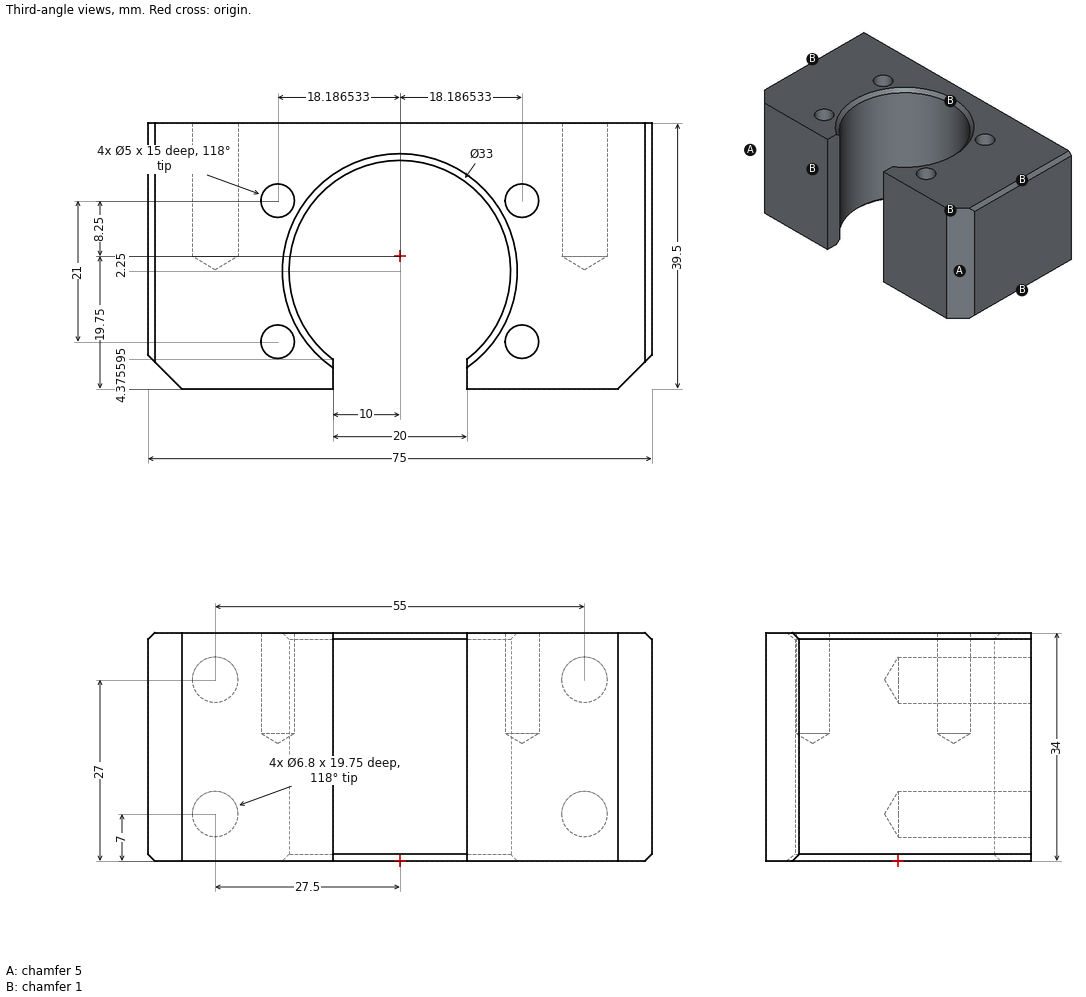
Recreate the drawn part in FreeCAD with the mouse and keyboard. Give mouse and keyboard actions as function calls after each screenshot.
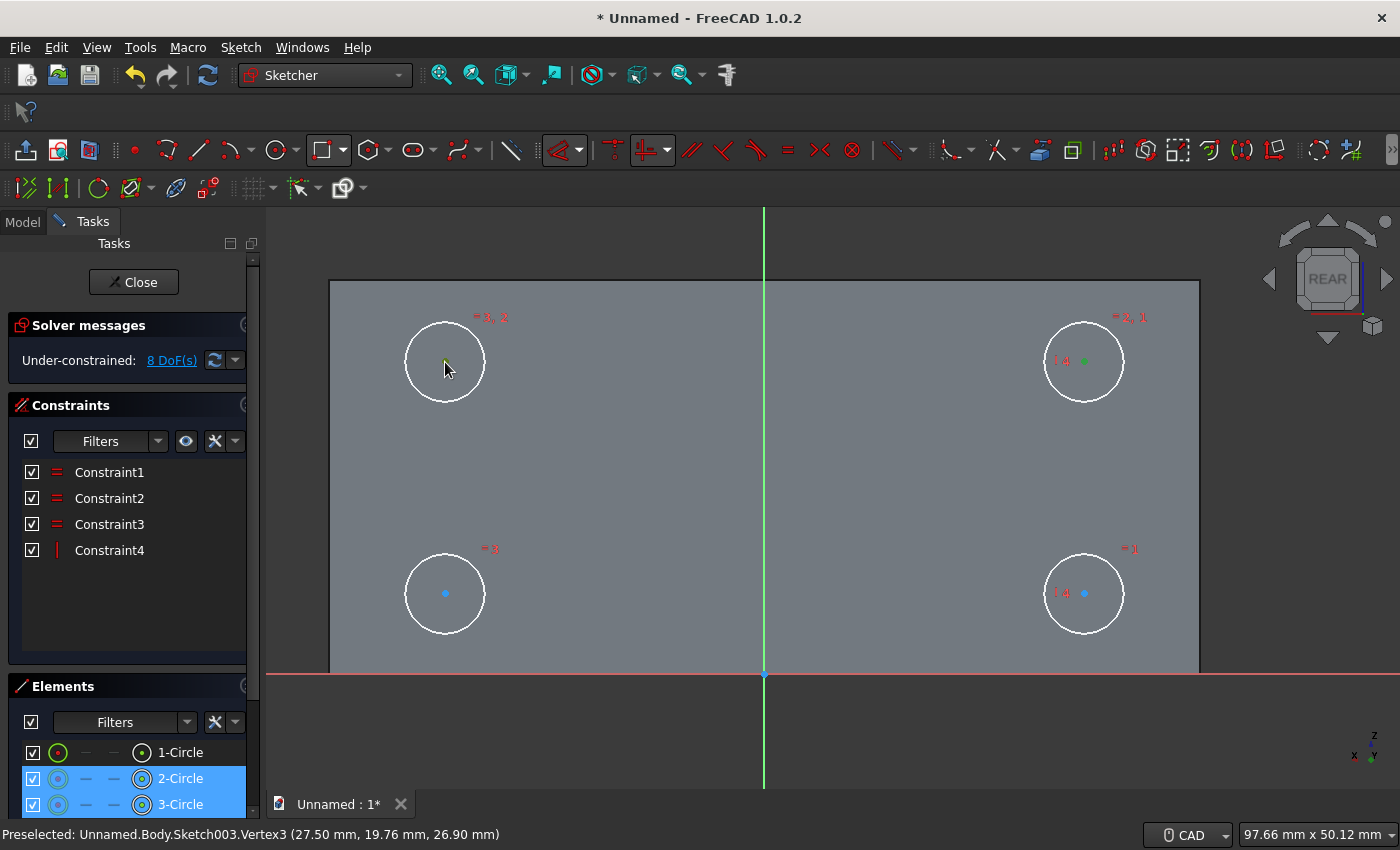
key(h)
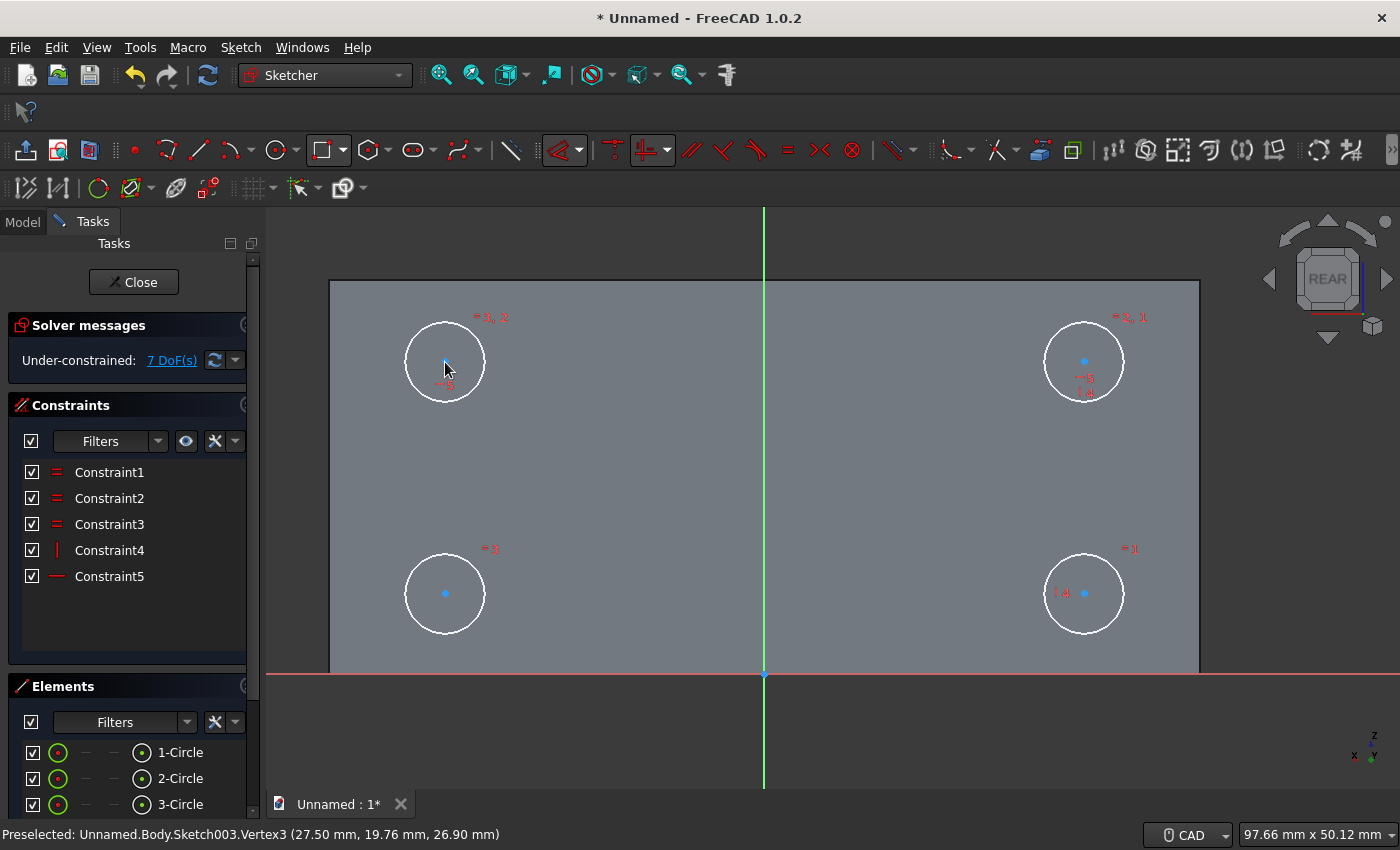
click(445, 362)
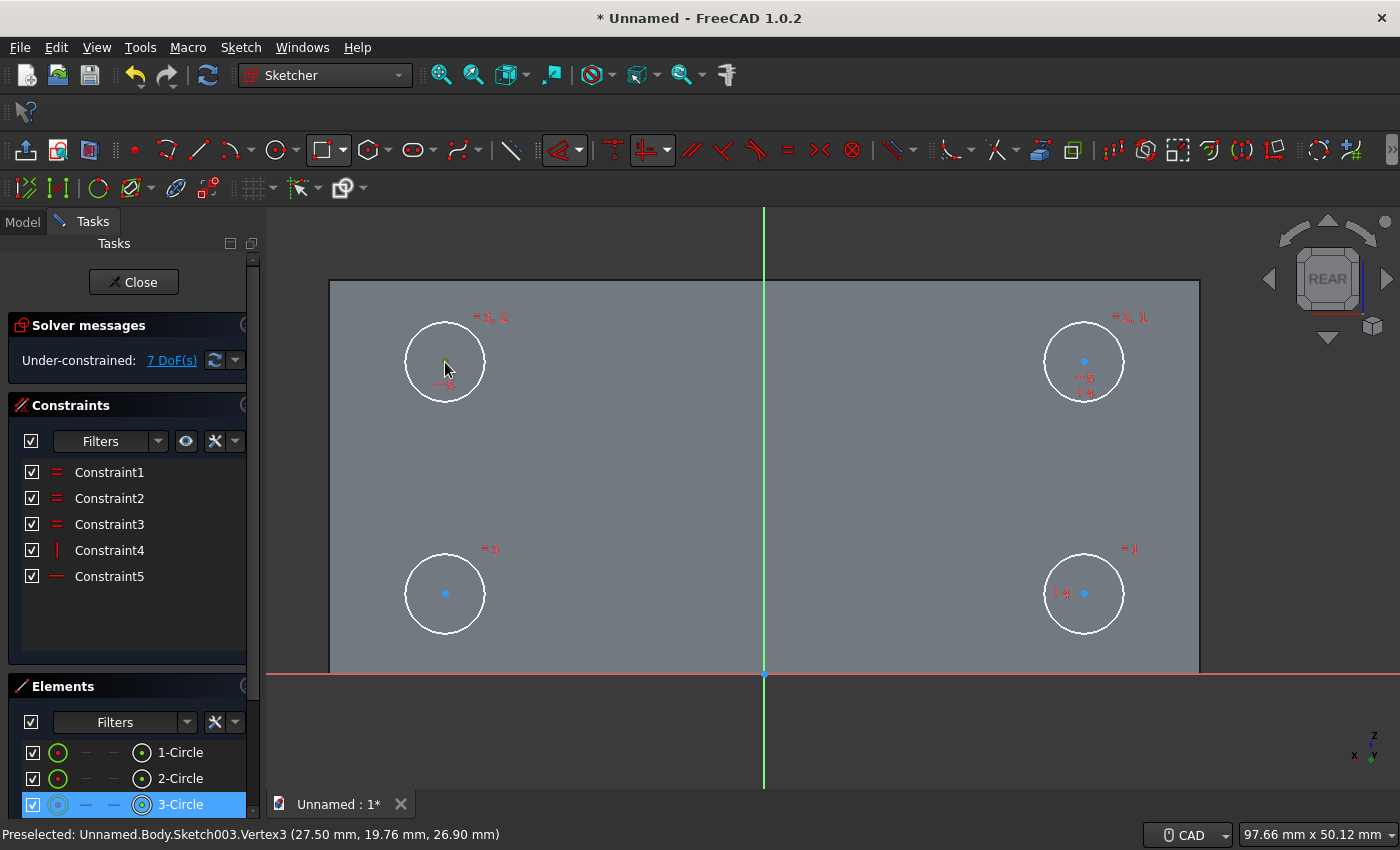
click(445, 594)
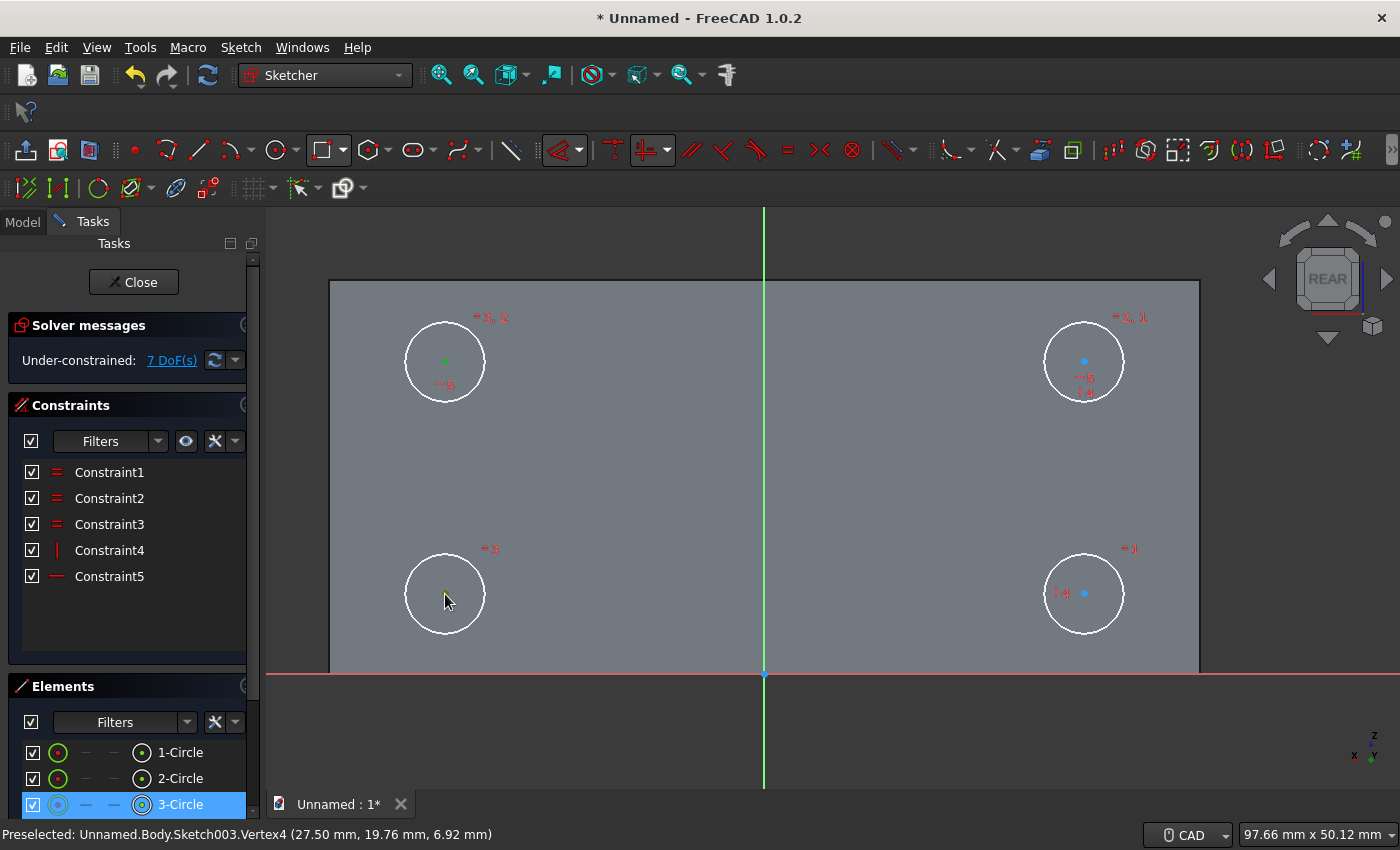
key(v)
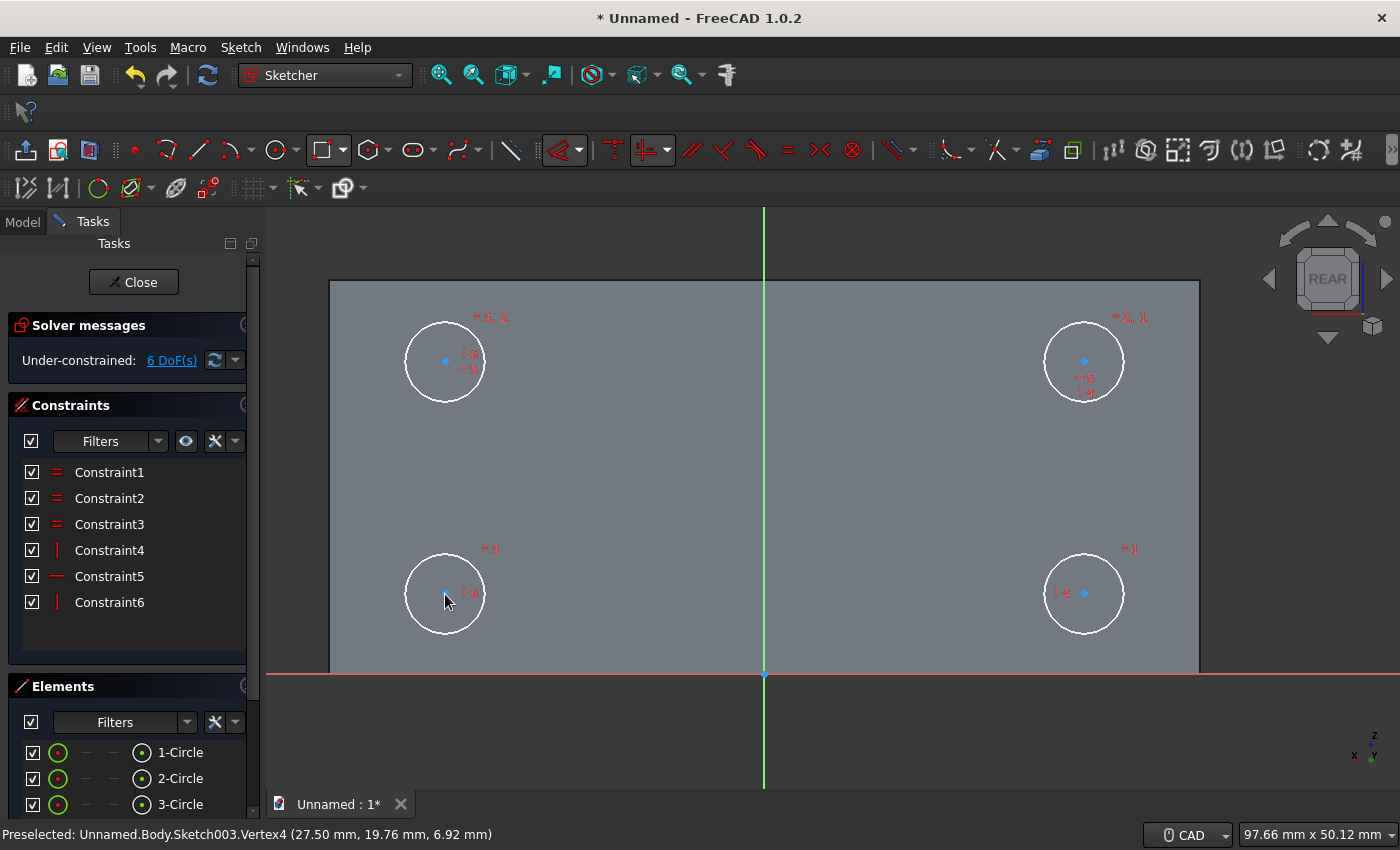
click(1084, 594)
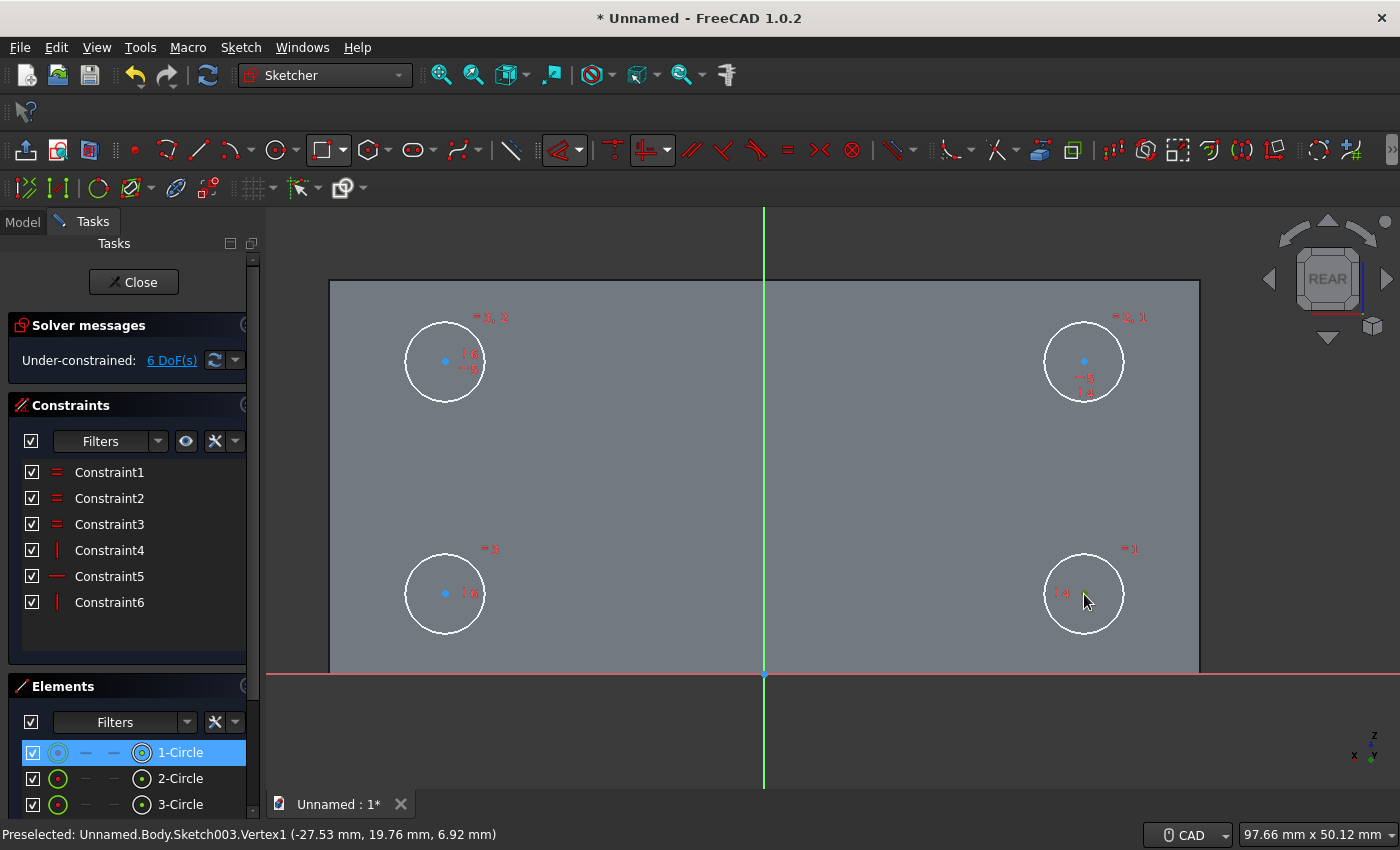
click(445, 594)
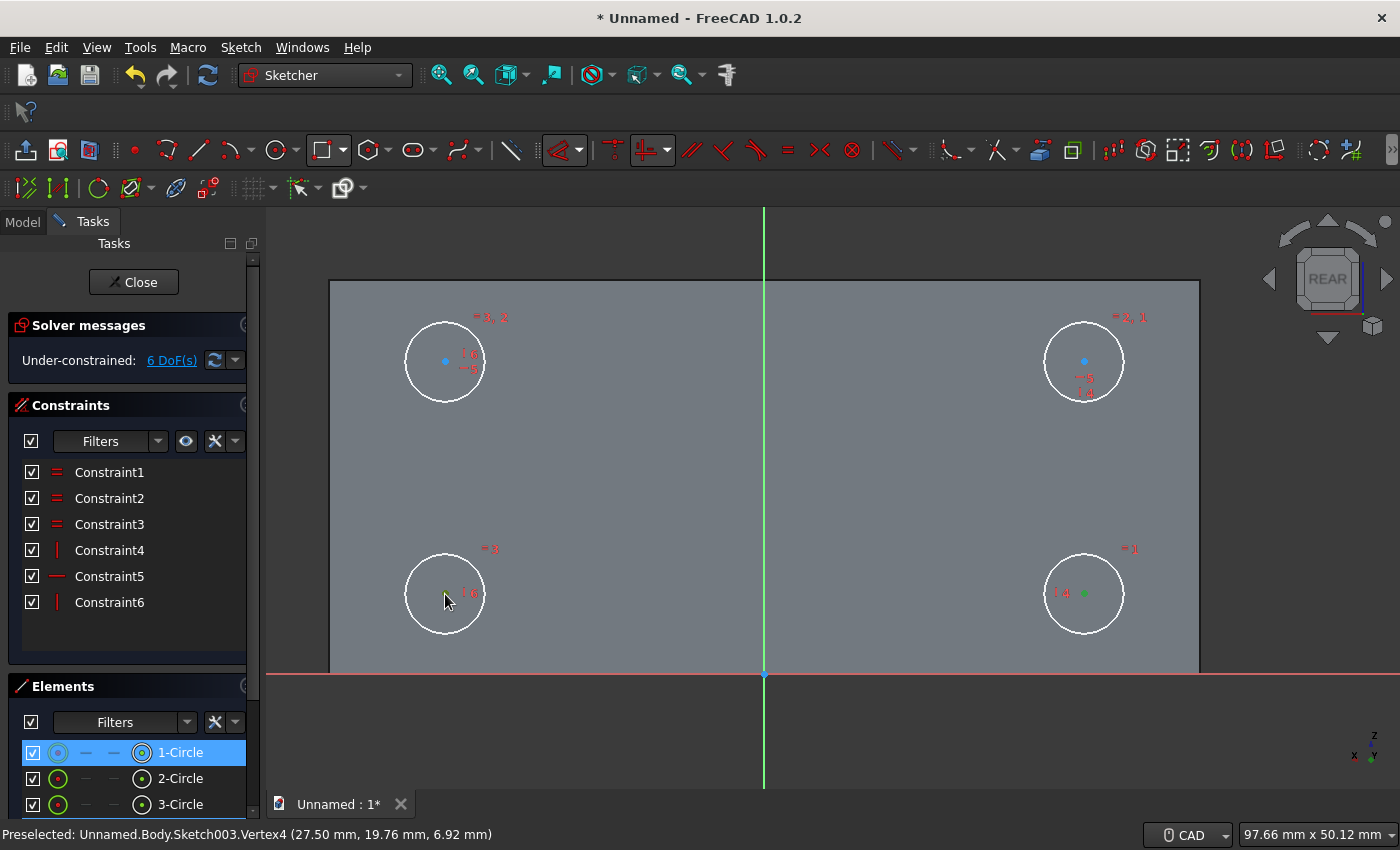
key(h)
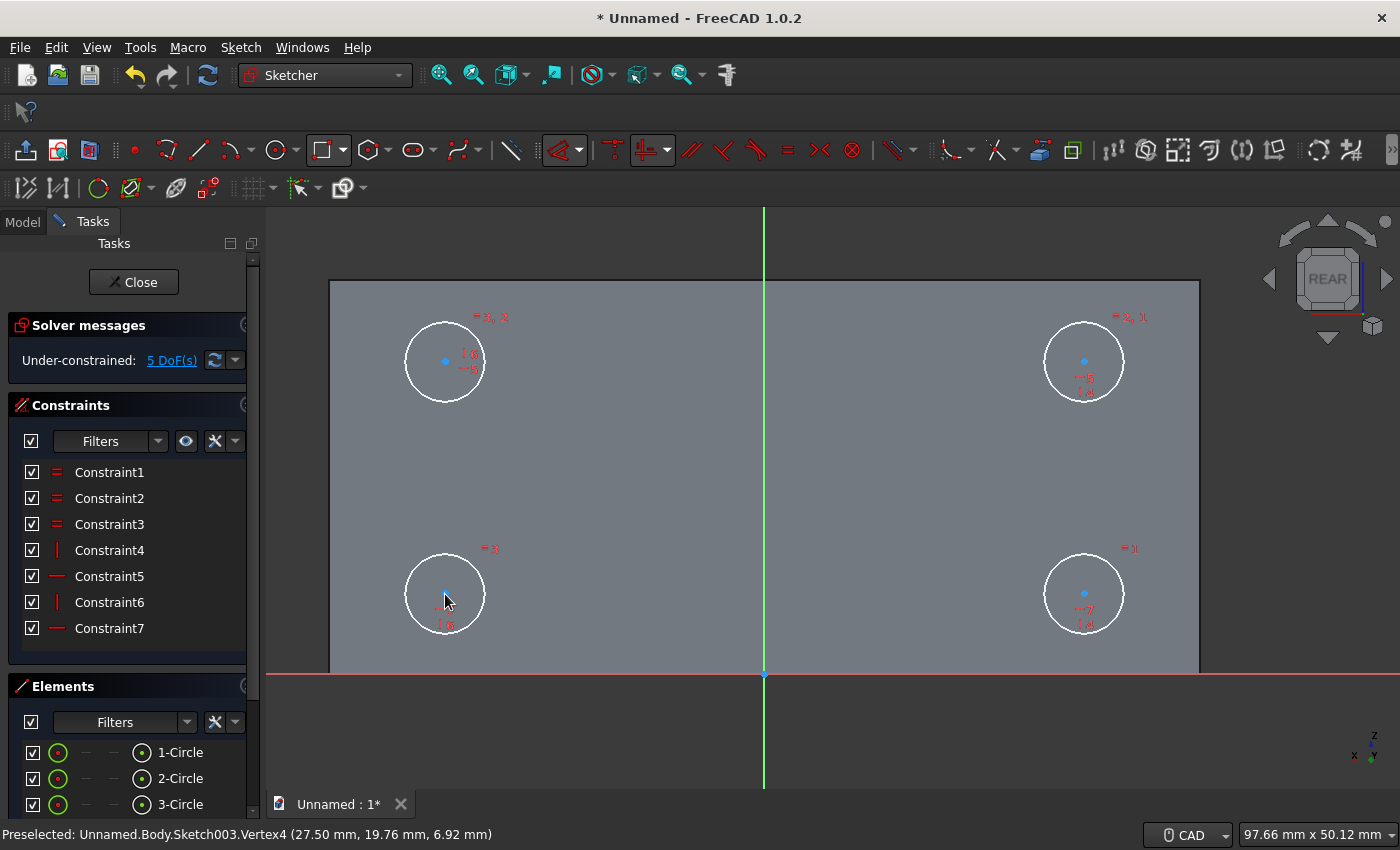
click(1112, 566)